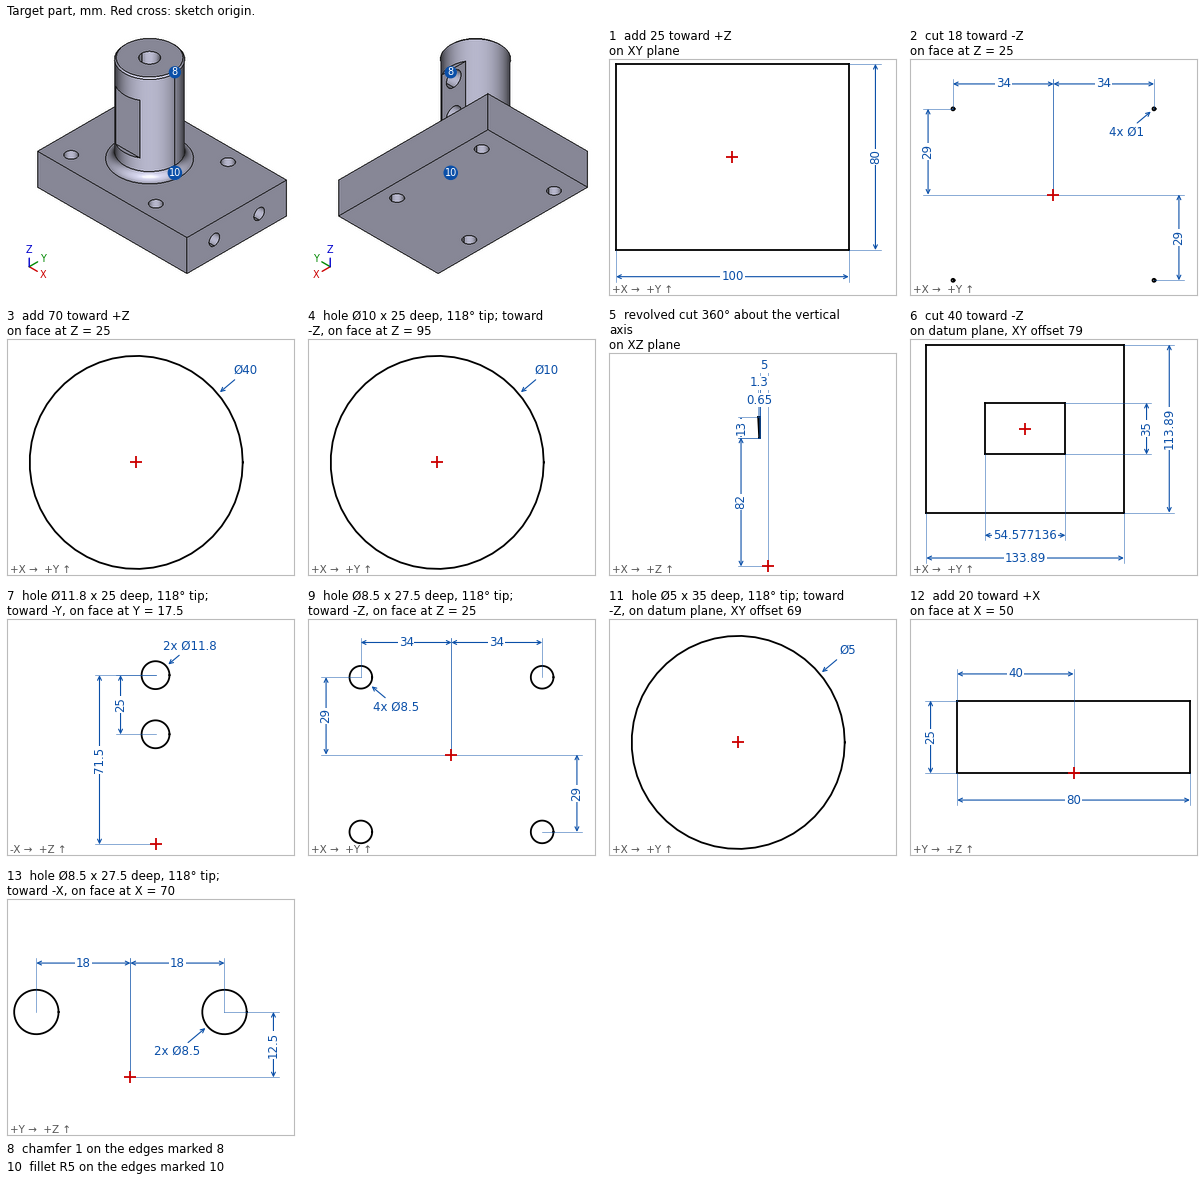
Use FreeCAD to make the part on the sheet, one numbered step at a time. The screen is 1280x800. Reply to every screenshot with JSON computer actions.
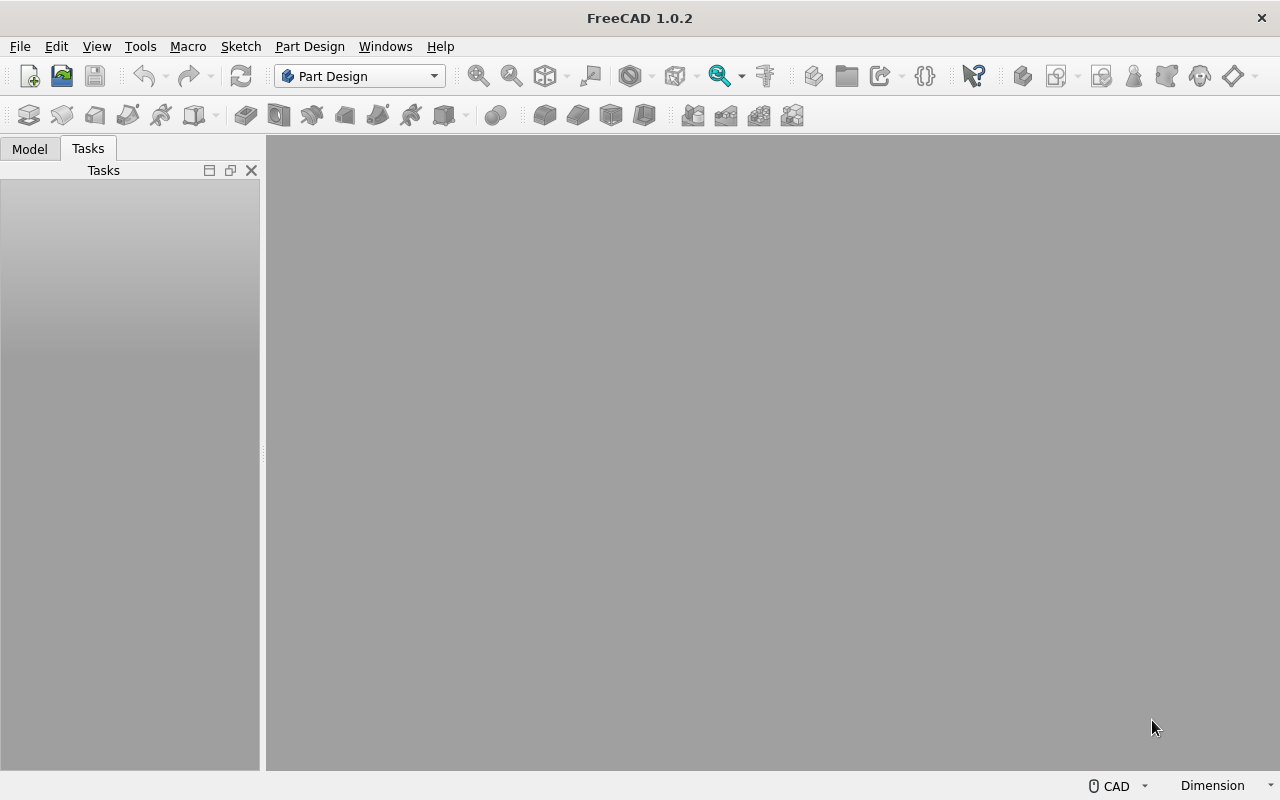
{"action": "key", "text": "ctrl+n"}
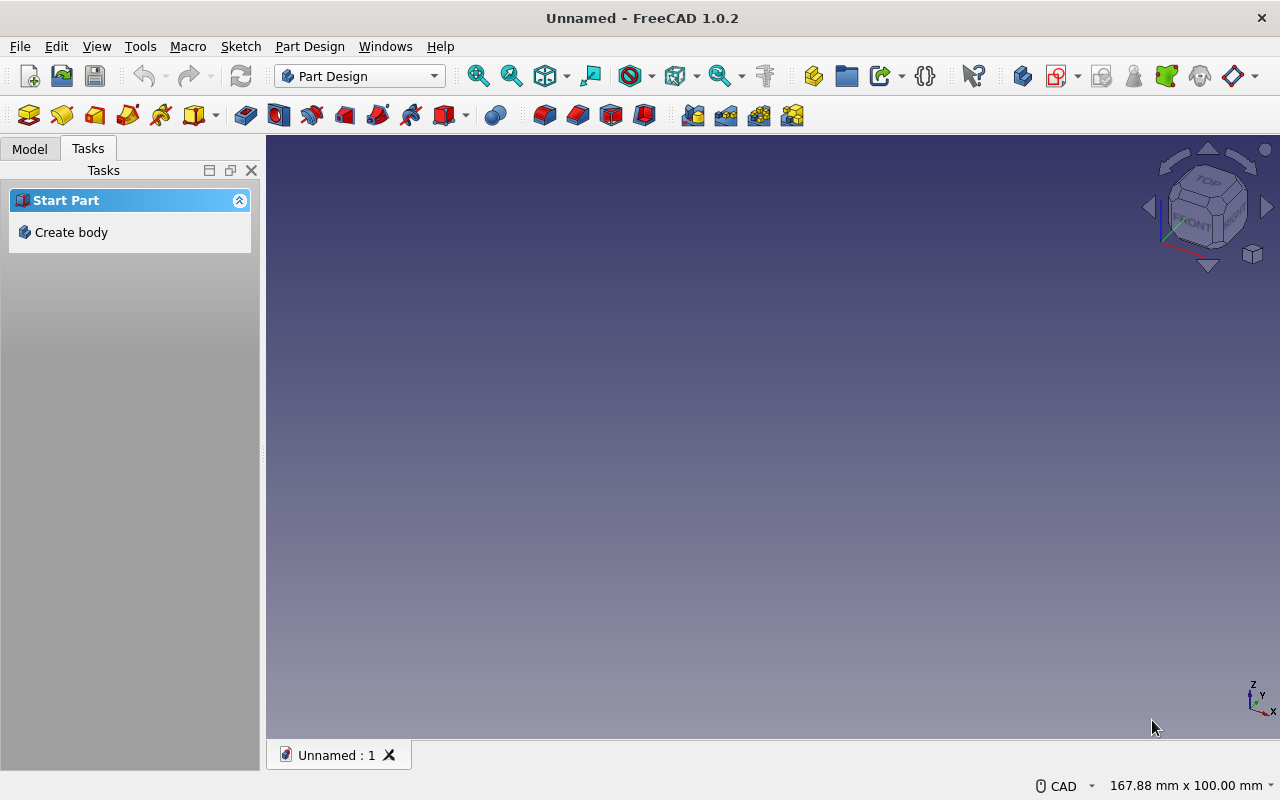
{"action": "left_click", "coordinate": [1056, 76]}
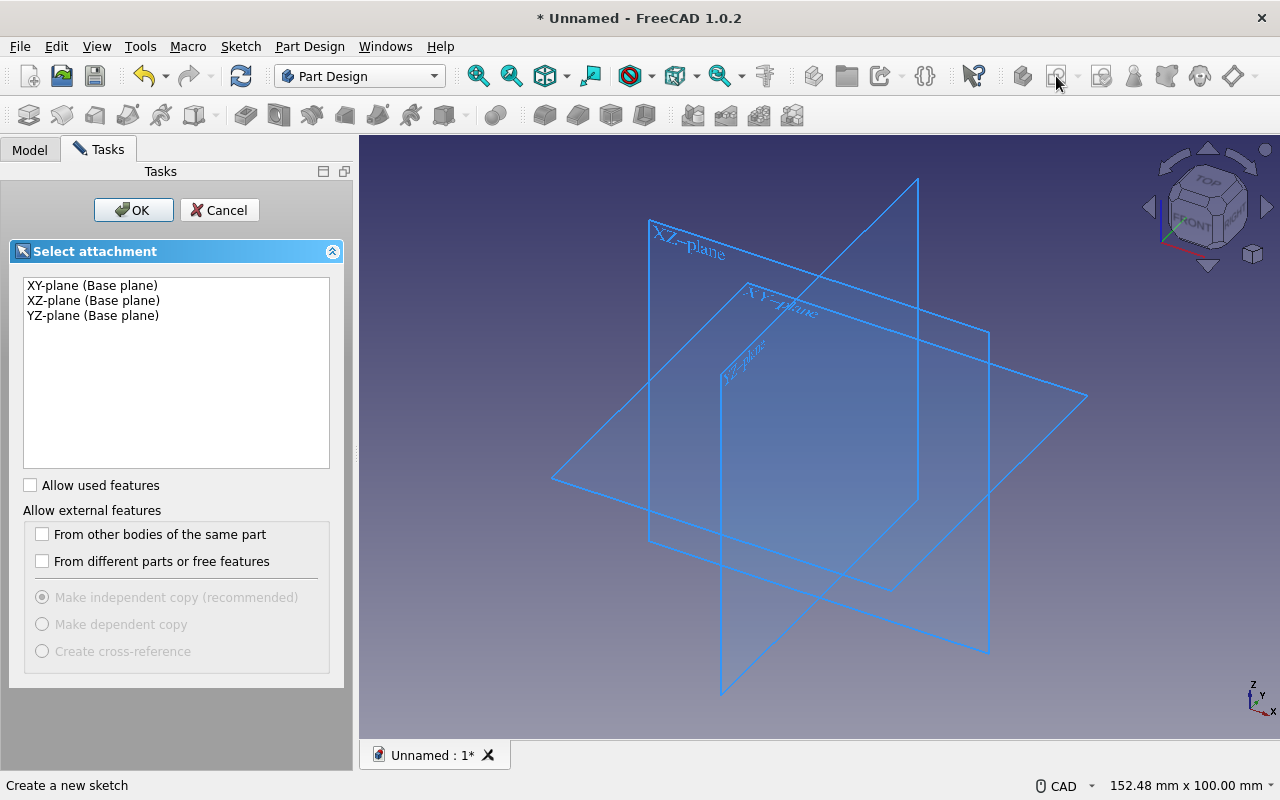
{"action": "left_click", "coordinate": [84, 286]}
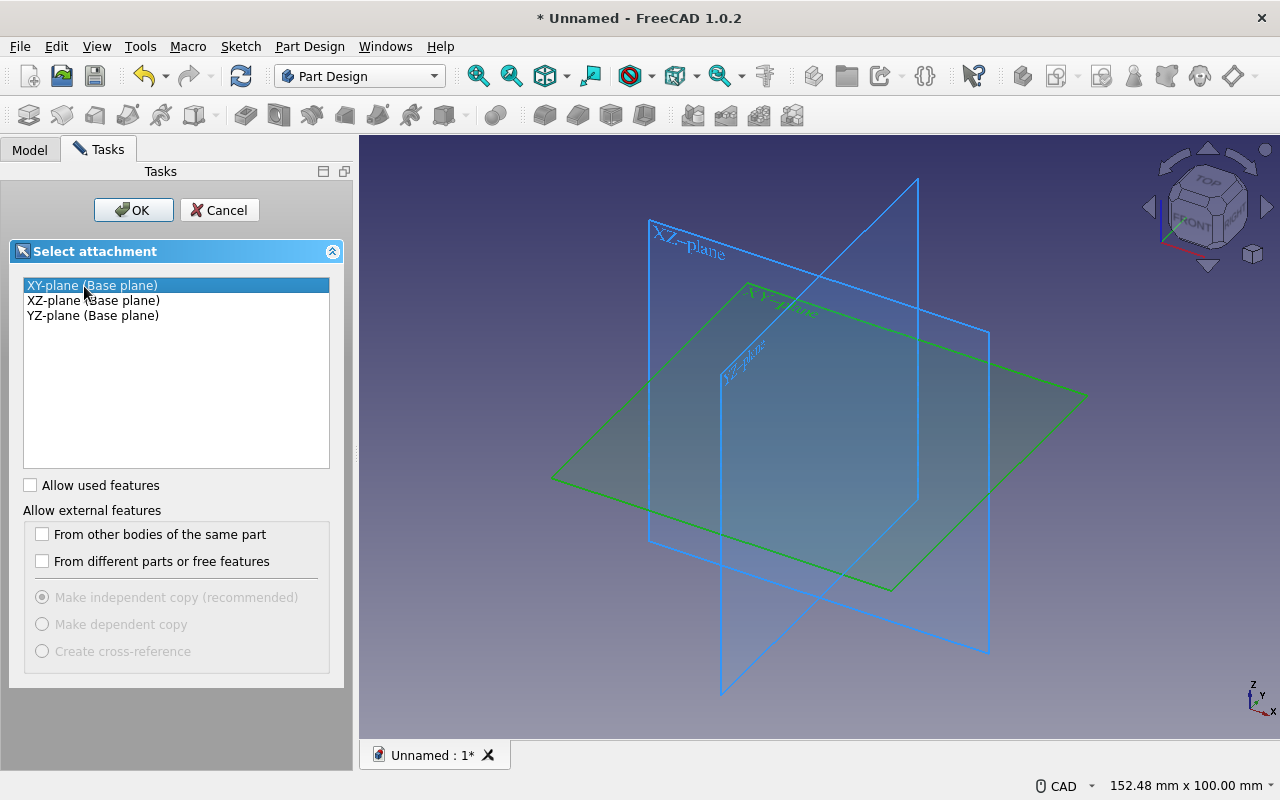
{"action": "left_click", "coordinate": [134, 210]}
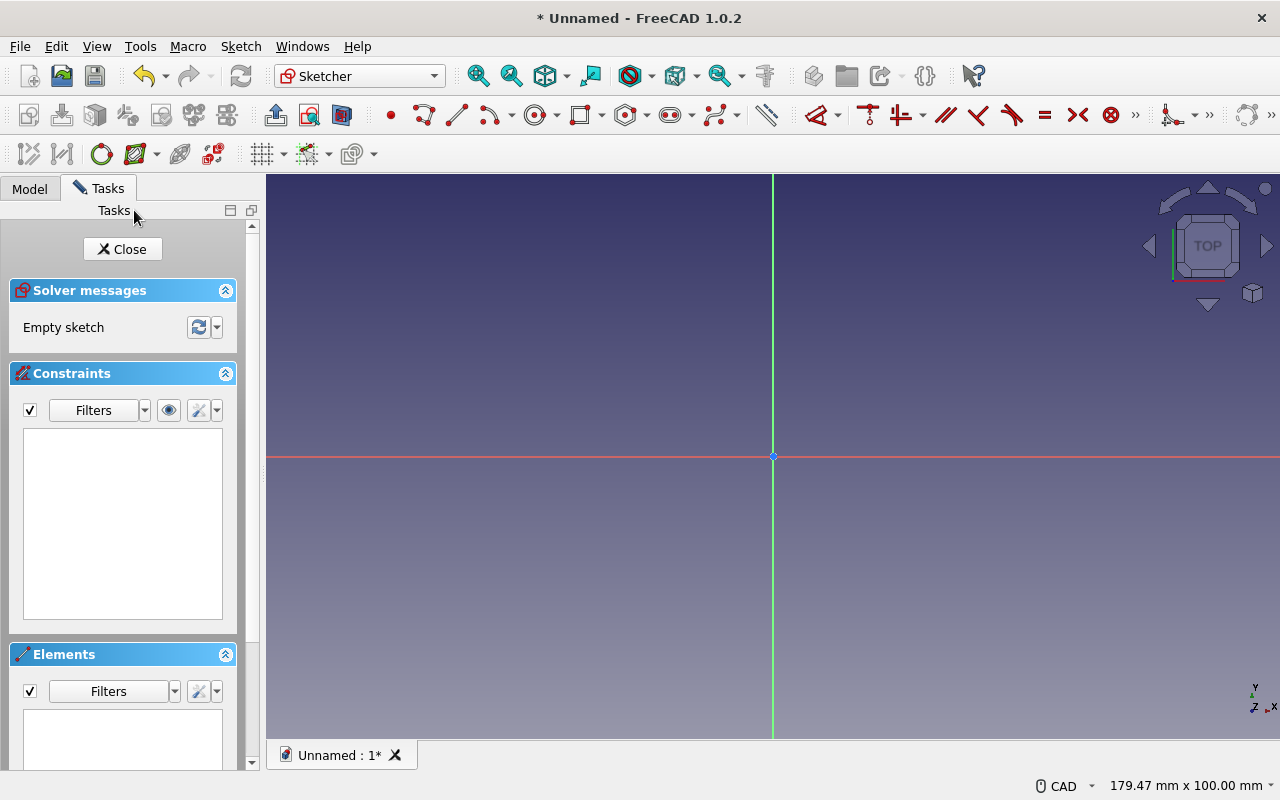
{"action": "key", "text": "g v"}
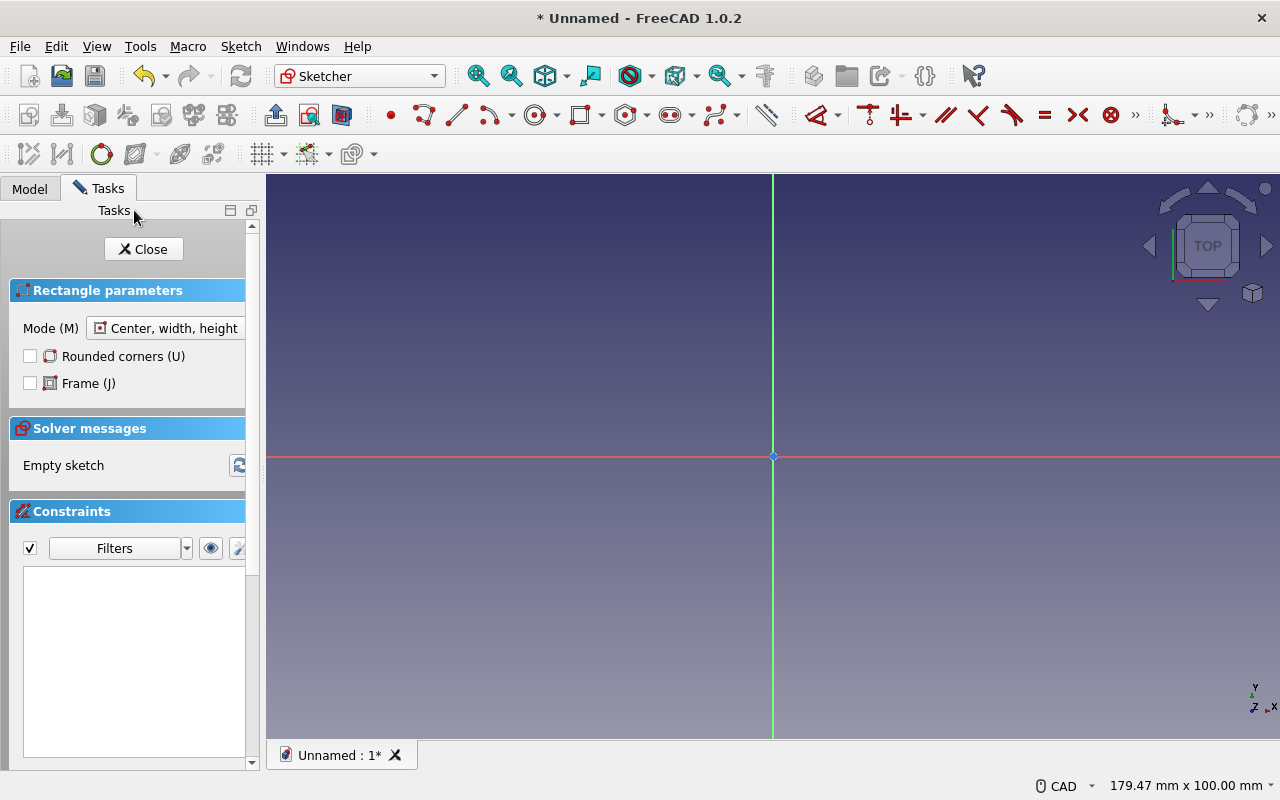
{"action": "left_click", "coordinate": [773, 456]}
{"action": "mouse_move", "coordinate": [1056, 230]}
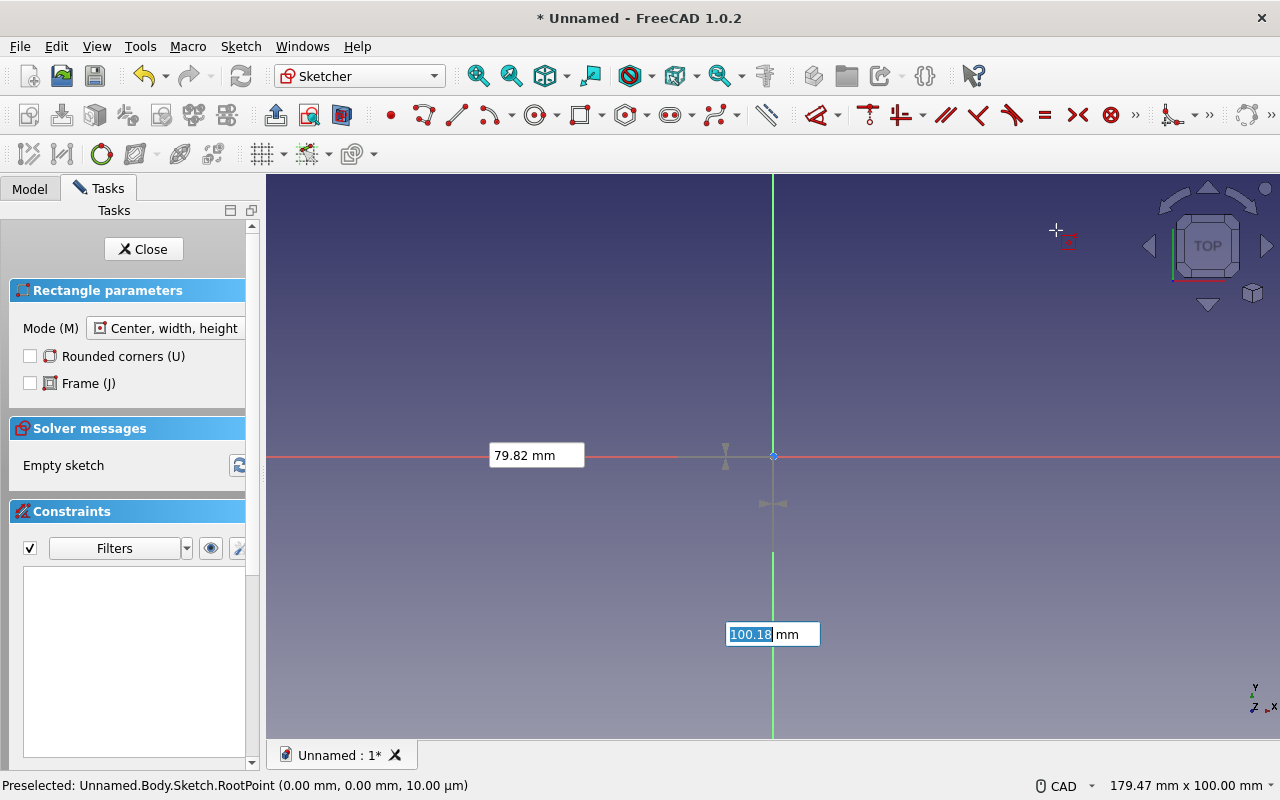
{"action": "type", "text": "100"}
{"action": "key", "text": "Tab"}
{"action": "type", "text": "80"}
{"action": "key", "text": "Return"}
{"action": "key", "text": "Escape"}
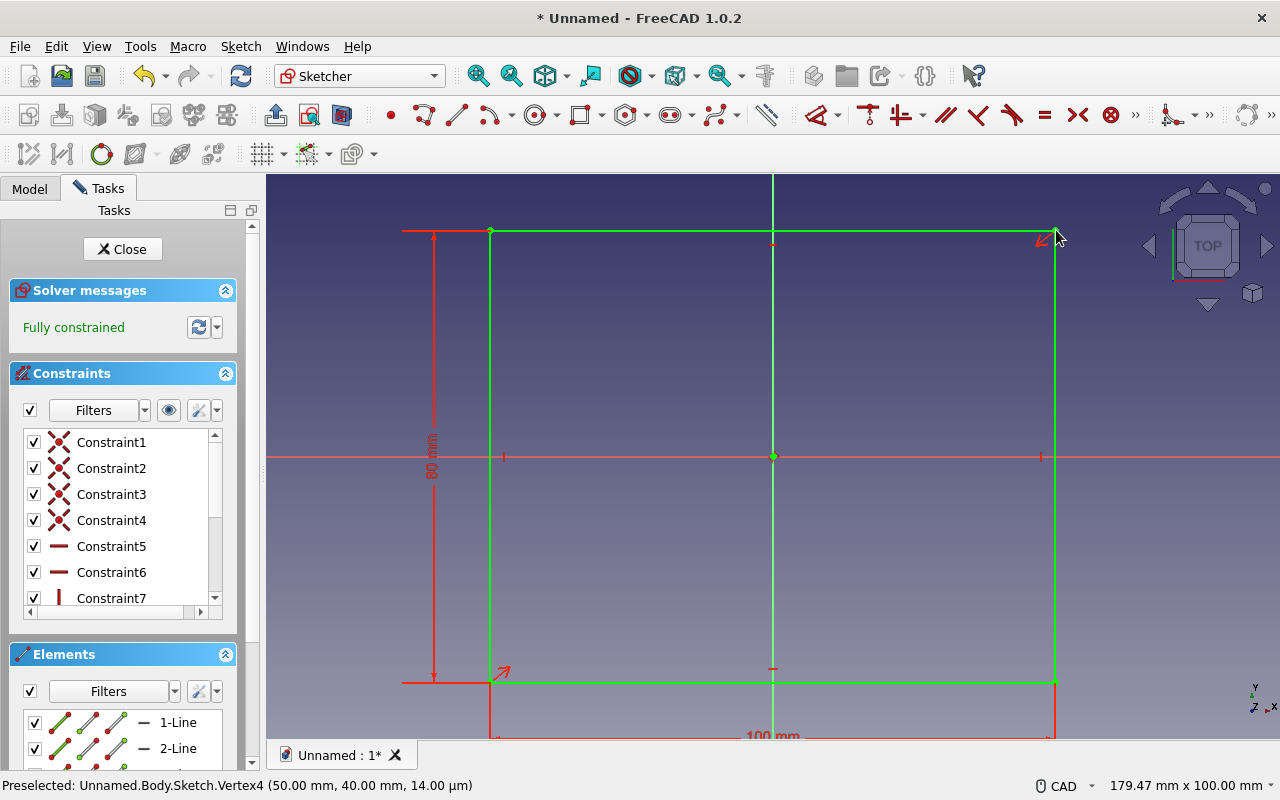
{"action": "left_click", "coordinate": [123, 249]}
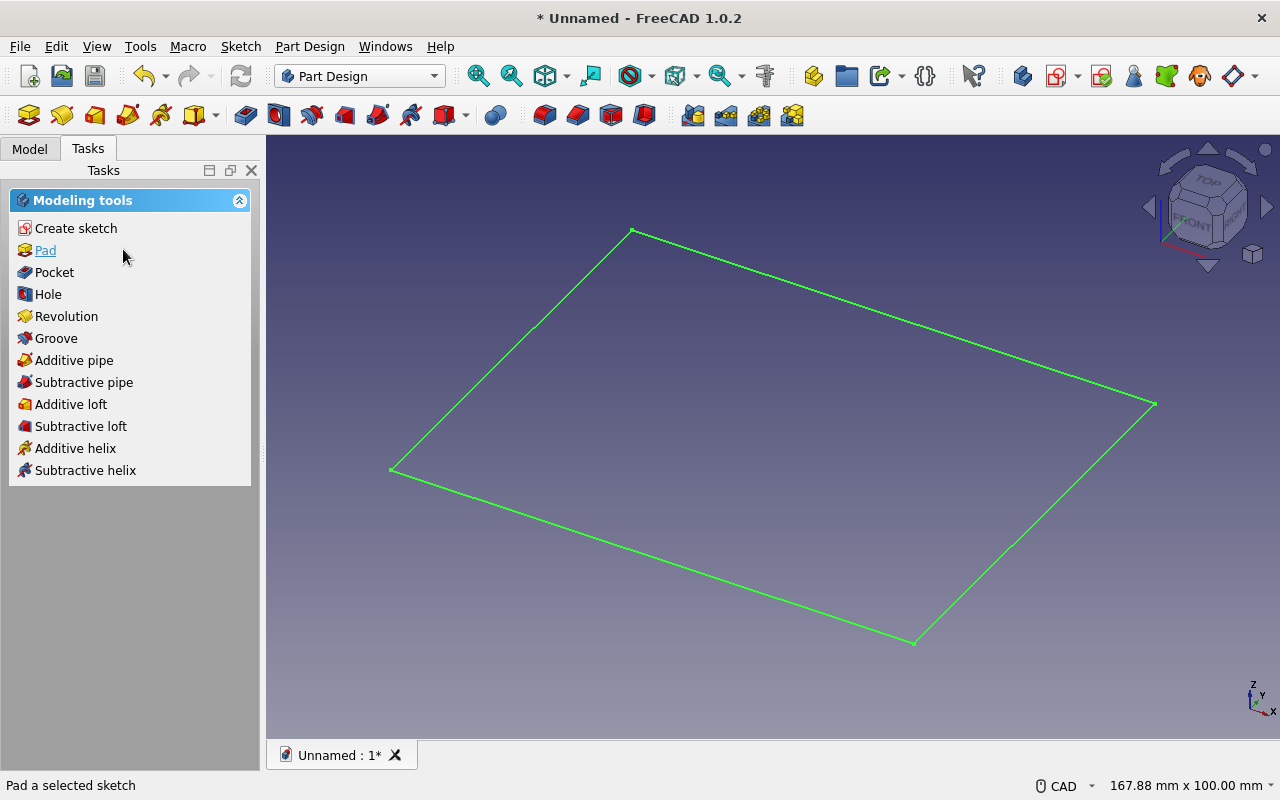
{"action": "left_click", "coordinate": [29, 116]}